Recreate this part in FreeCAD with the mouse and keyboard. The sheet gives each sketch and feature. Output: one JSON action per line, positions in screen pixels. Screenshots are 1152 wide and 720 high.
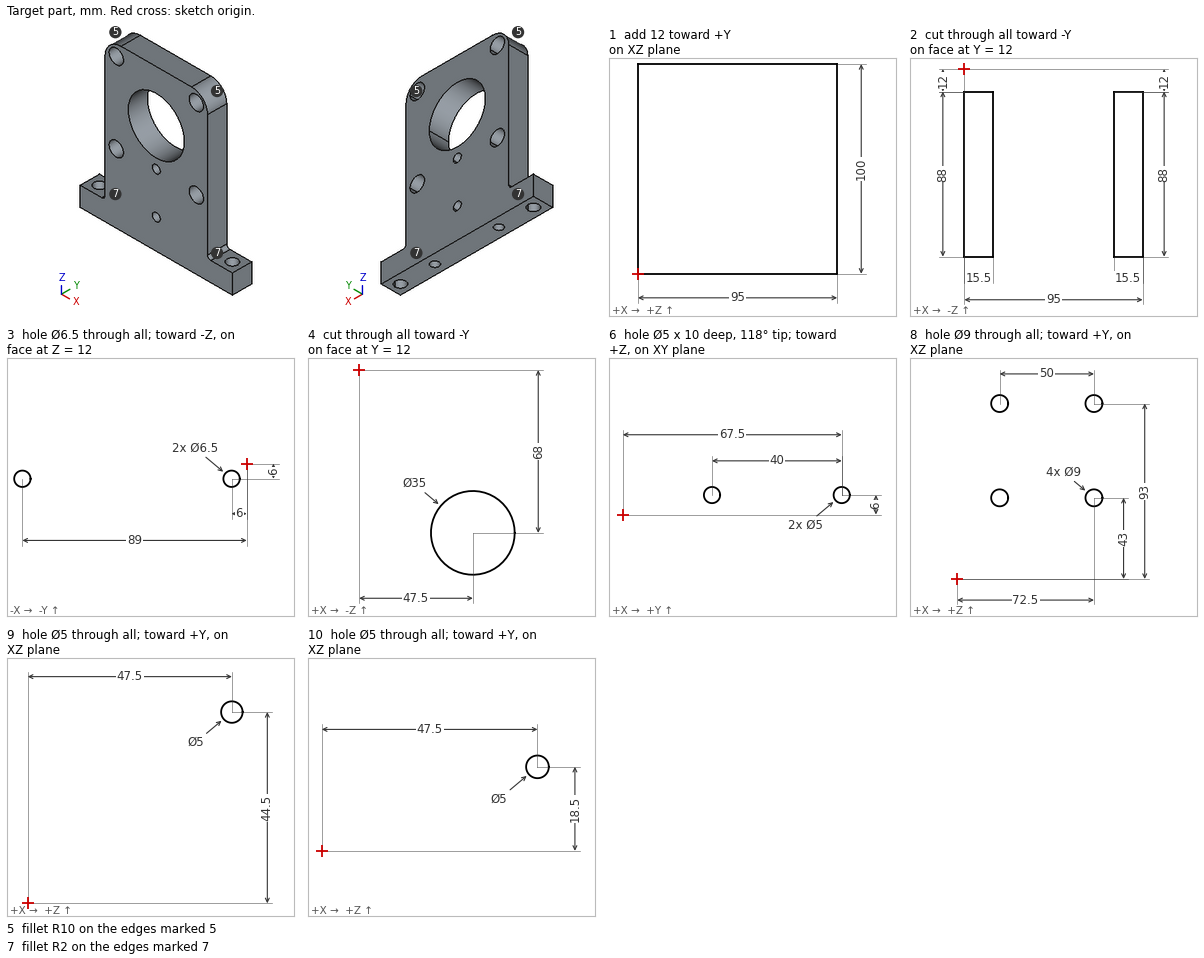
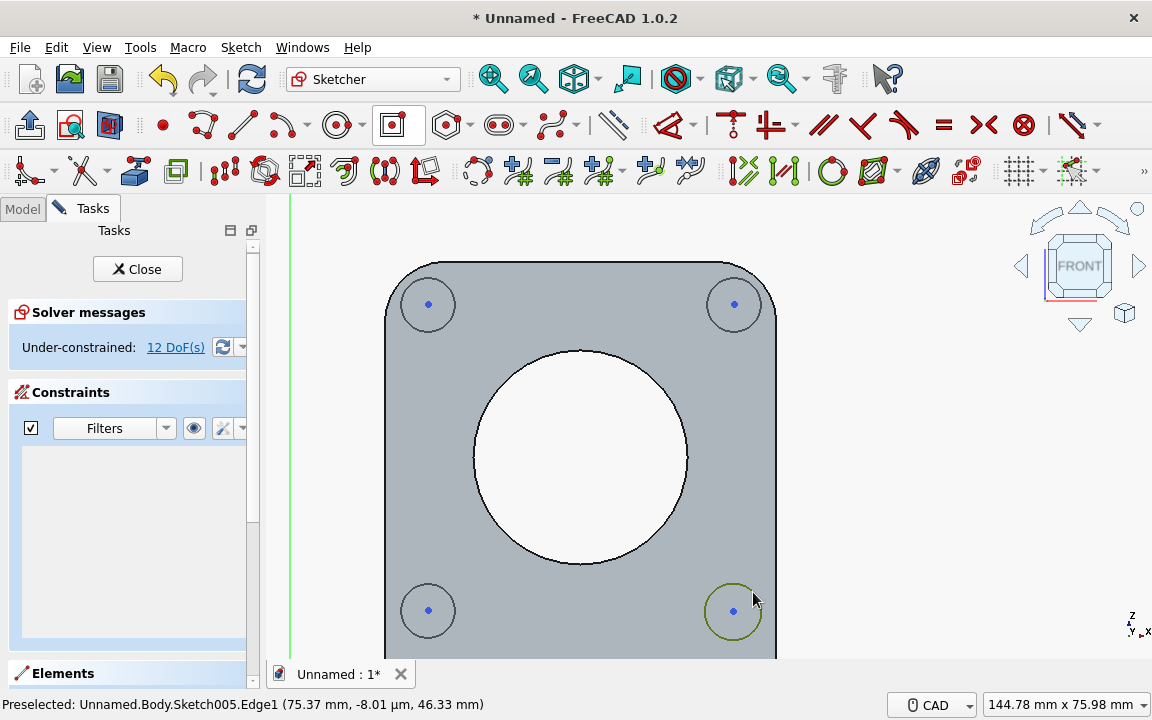
{"action": "left_click", "coordinate": [753, 286]}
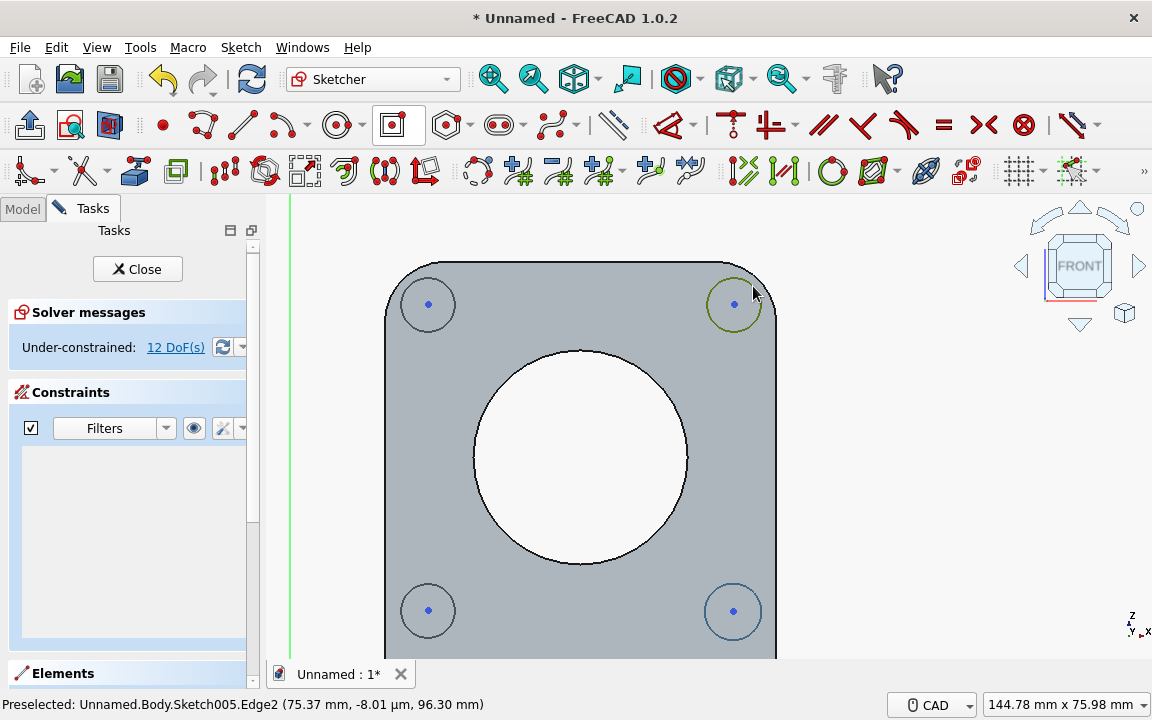
{"action": "left_click", "coordinate": [447, 286]}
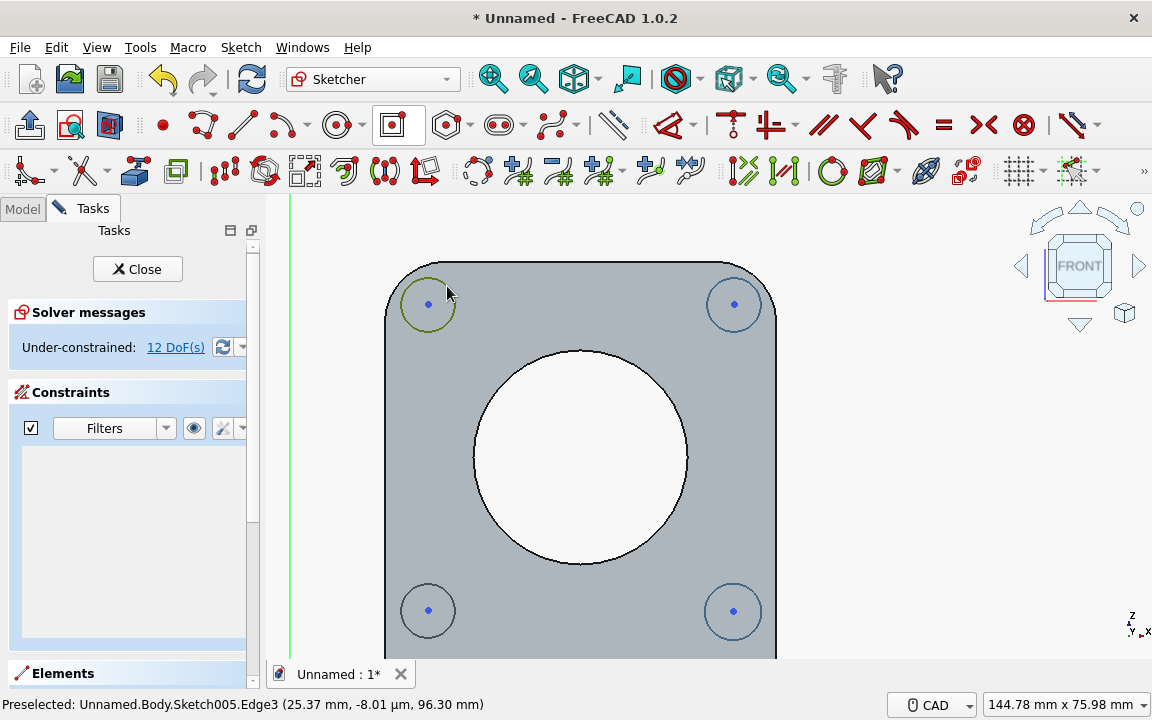
{"action": "left_click", "coordinate": [447, 592]}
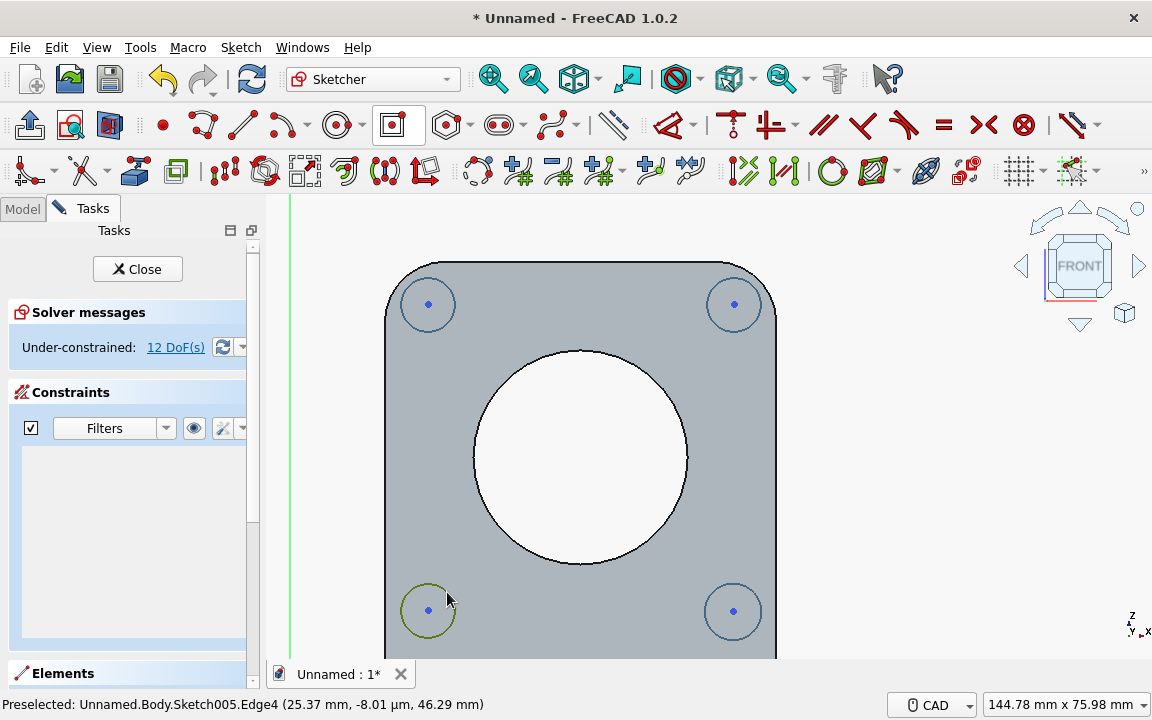
{"action": "left_click", "coordinate": [944, 126]}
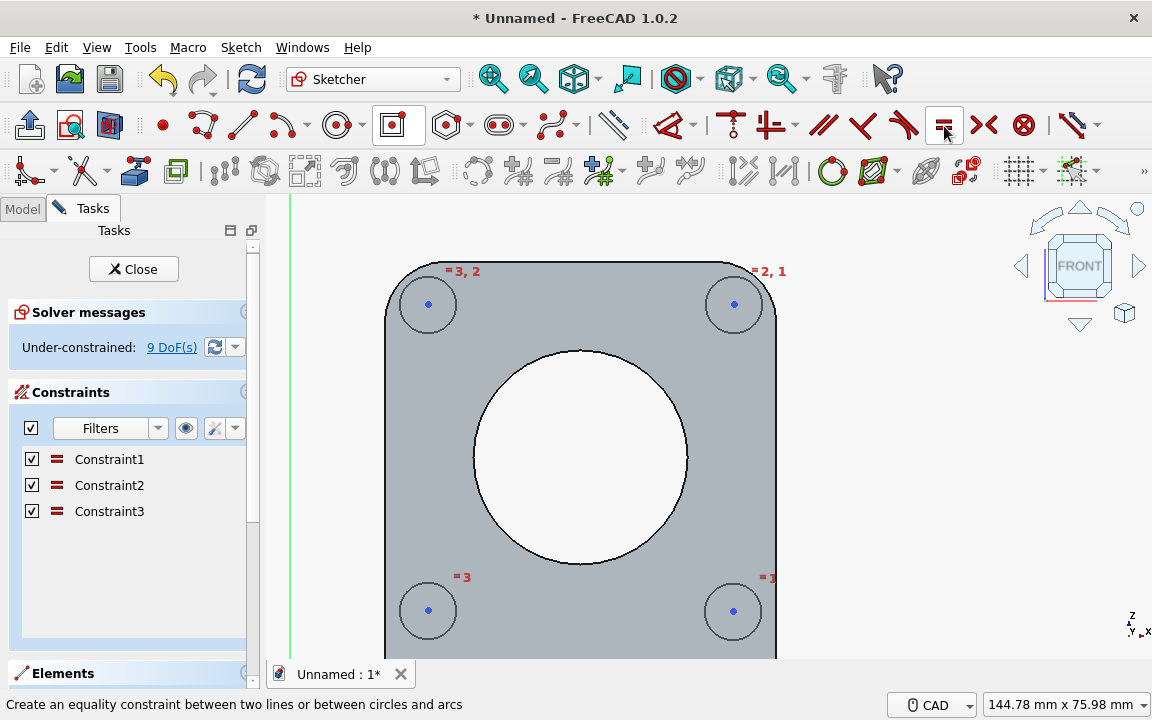
{"action": "left_click", "coordinate": [733, 612]}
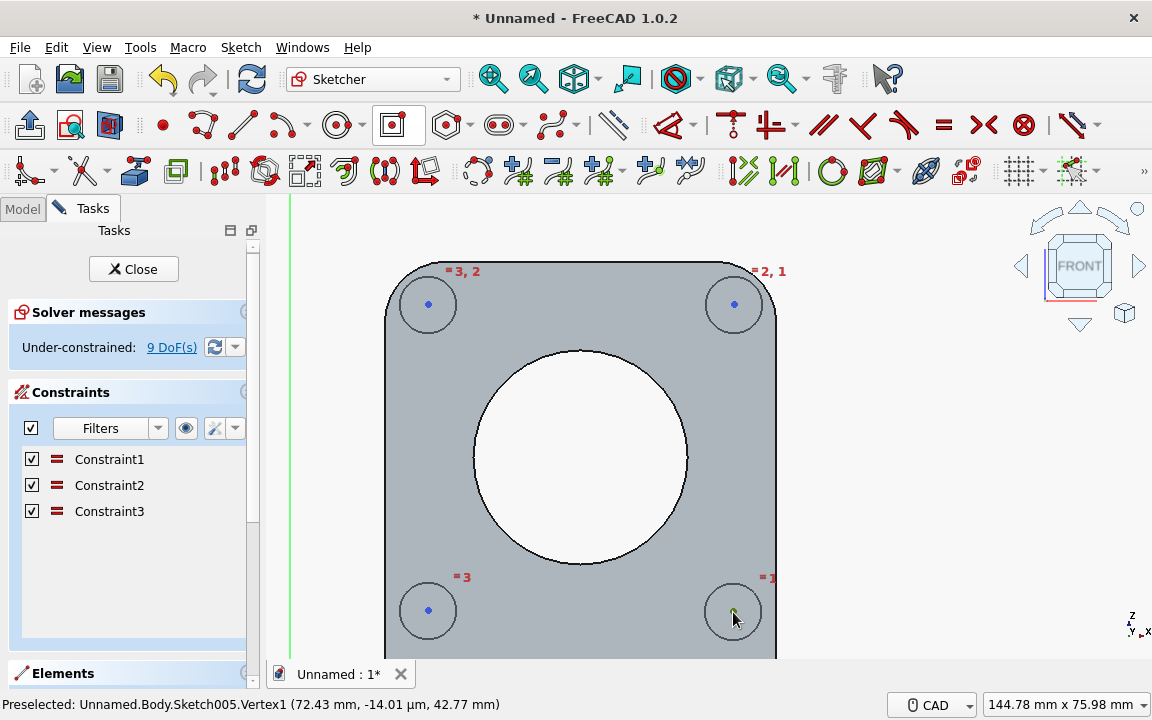
{"action": "left_click", "coordinate": [734, 305]}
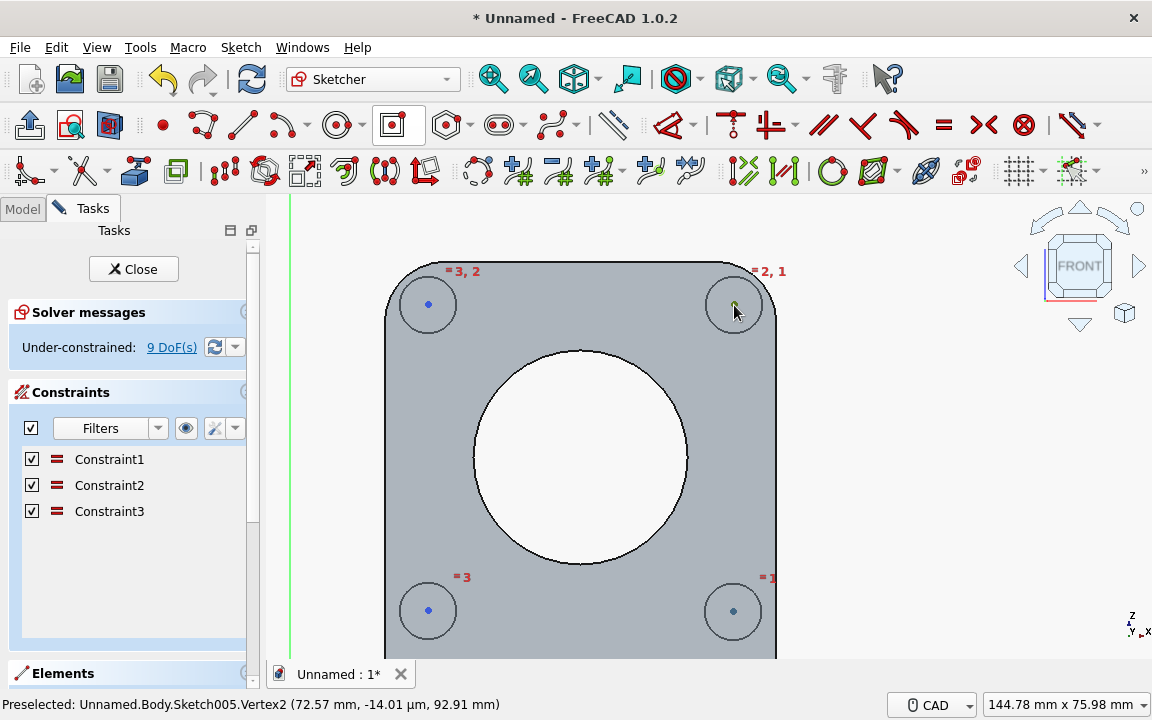
{"action": "left_click", "coordinate": [798, 126]}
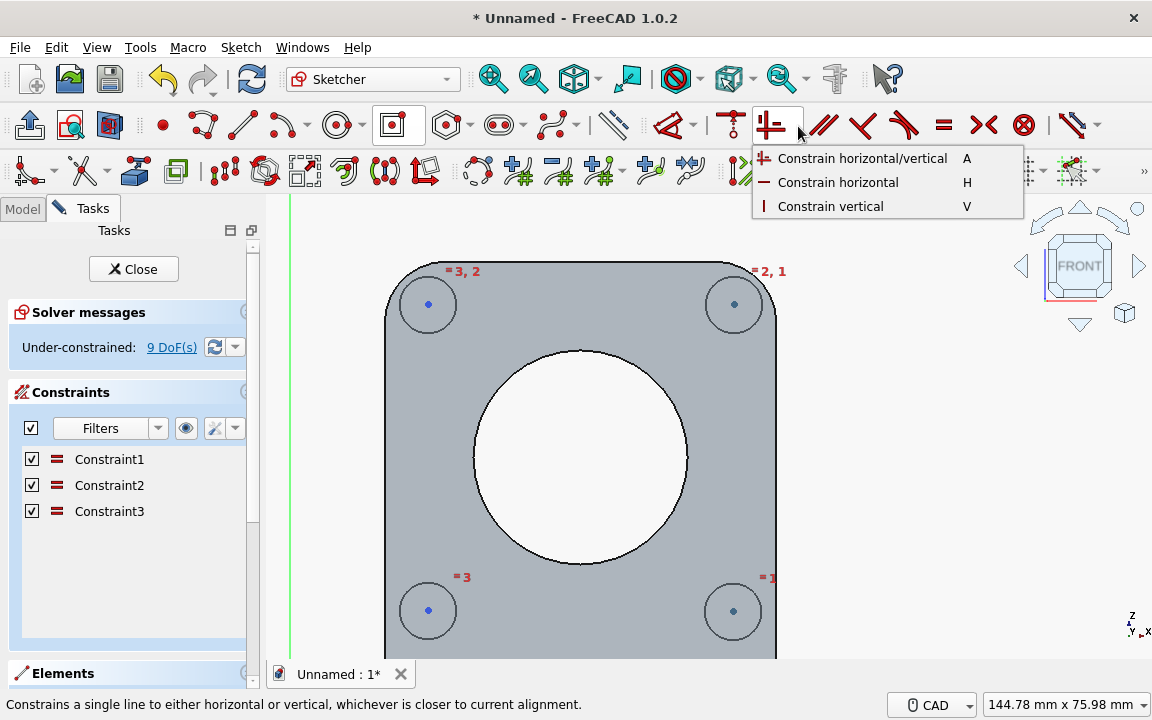
{"action": "left_click", "coordinate": [888, 206]}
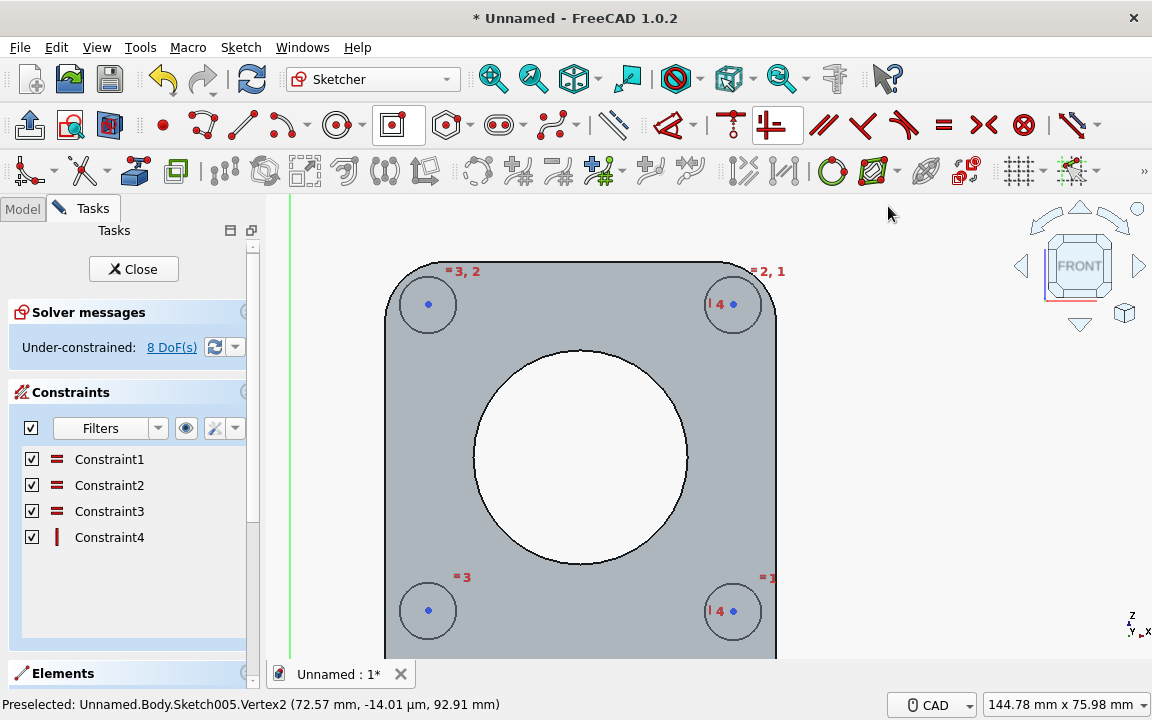
{"action": "left_click", "coordinate": [733, 305]}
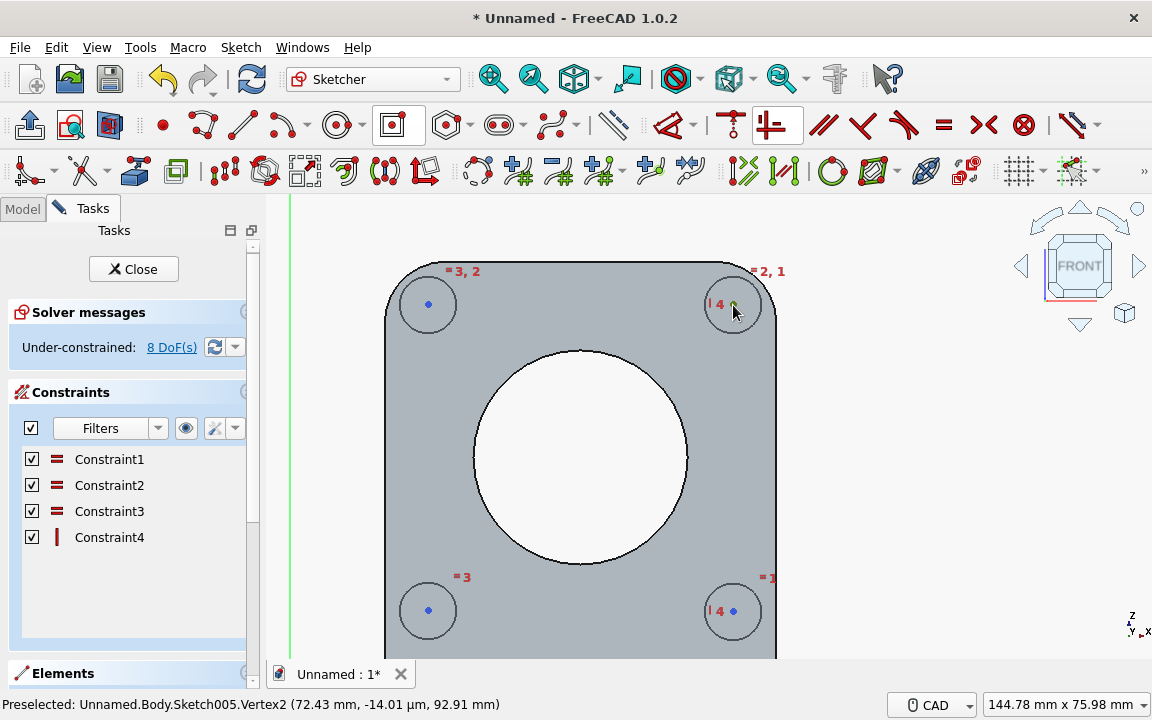
{"action": "left_click", "coordinate": [428, 305]}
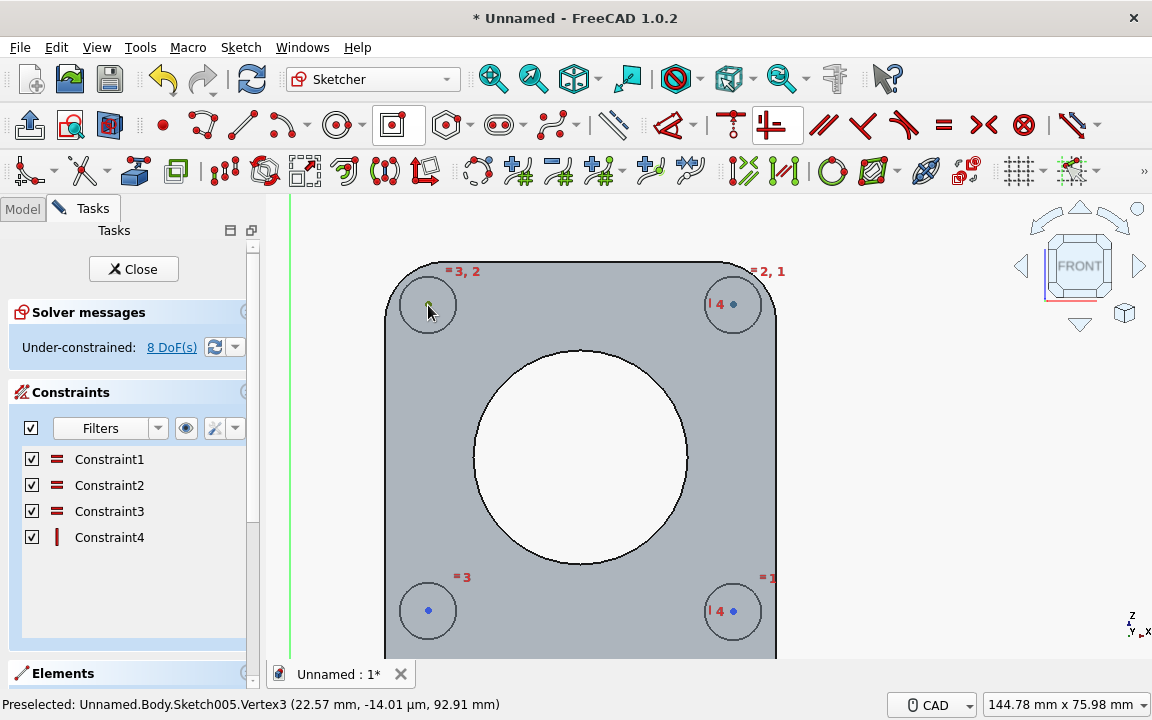
{"action": "left_click", "coordinate": [798, 126]}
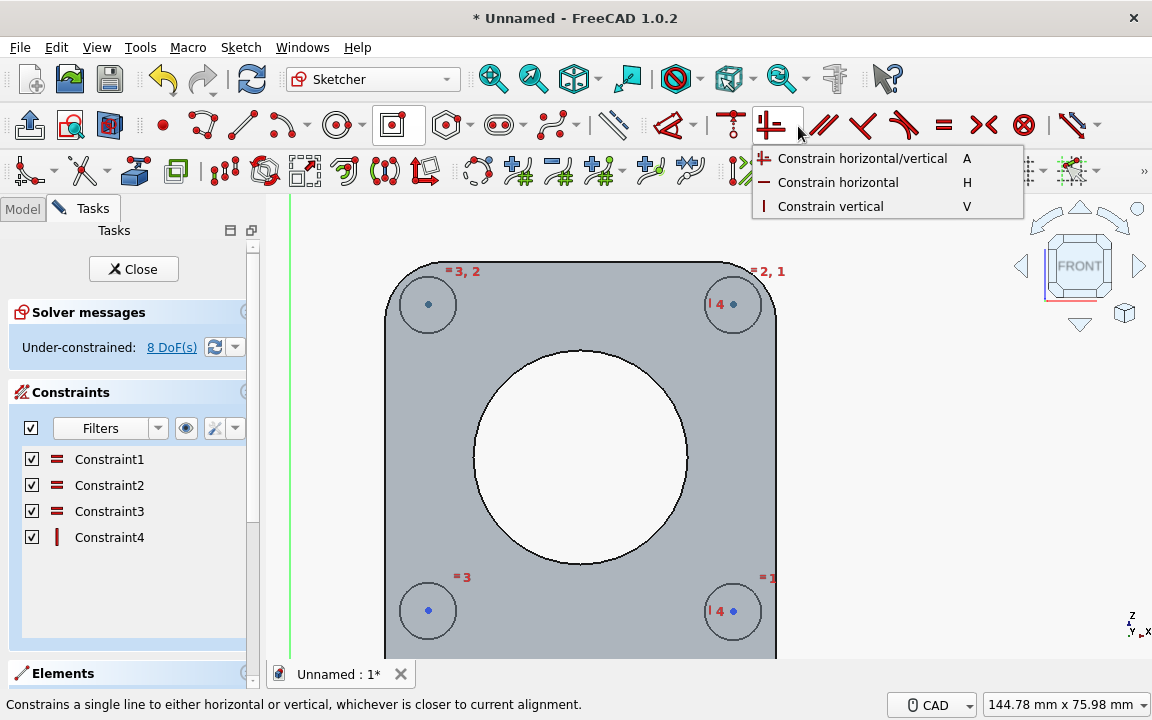
{"action": "left_click", "coordinate": [888, 182]}